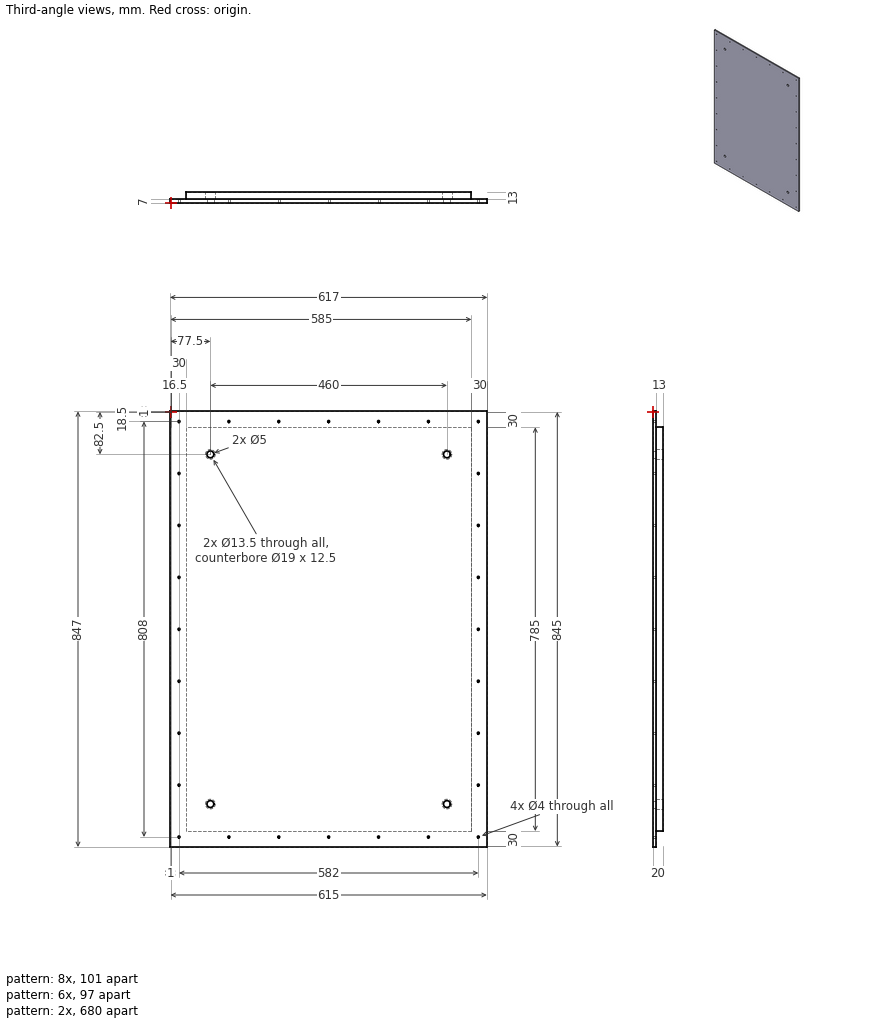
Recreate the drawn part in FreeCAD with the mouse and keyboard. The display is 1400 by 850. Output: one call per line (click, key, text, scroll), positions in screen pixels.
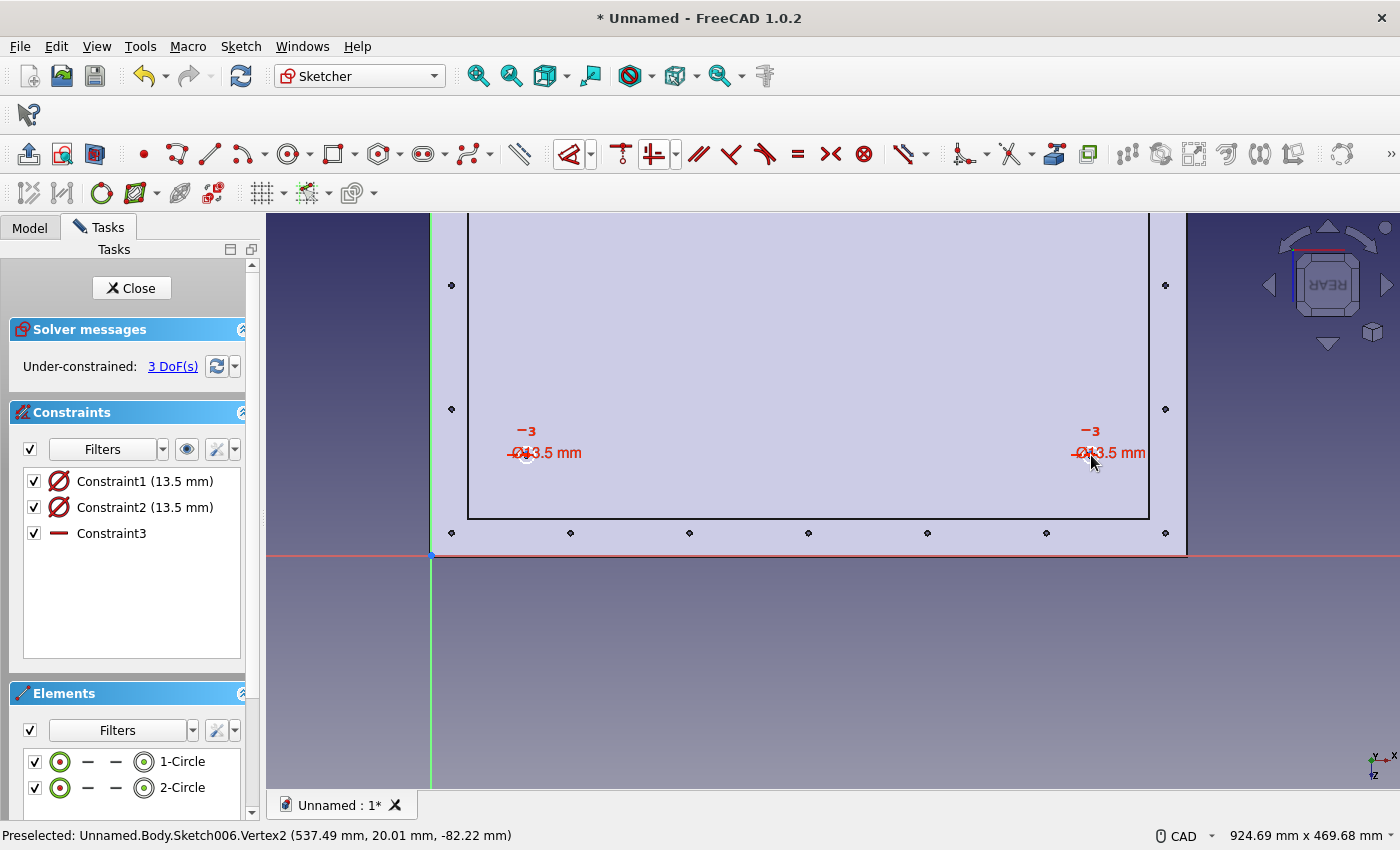
click(527, 455)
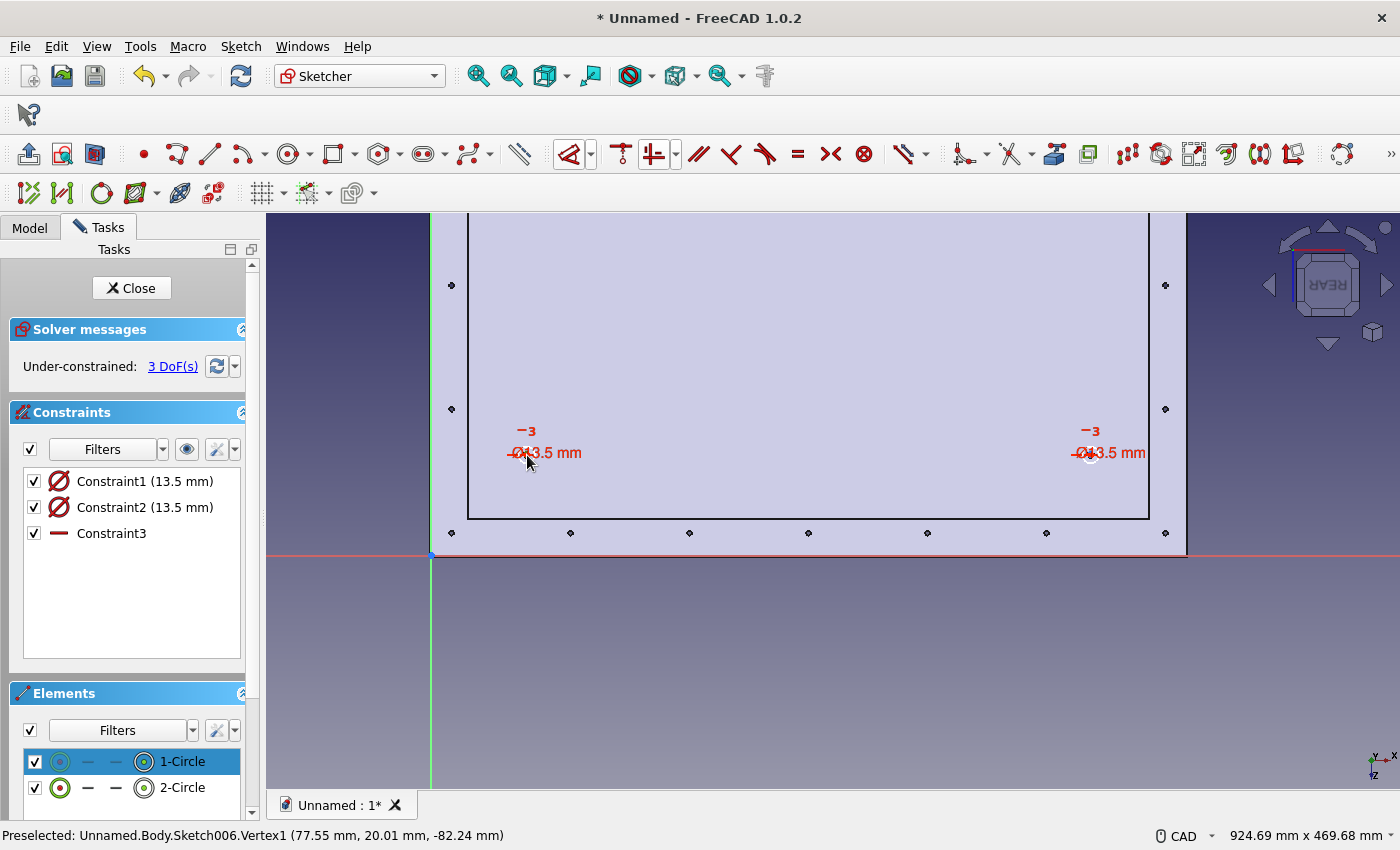
key(l)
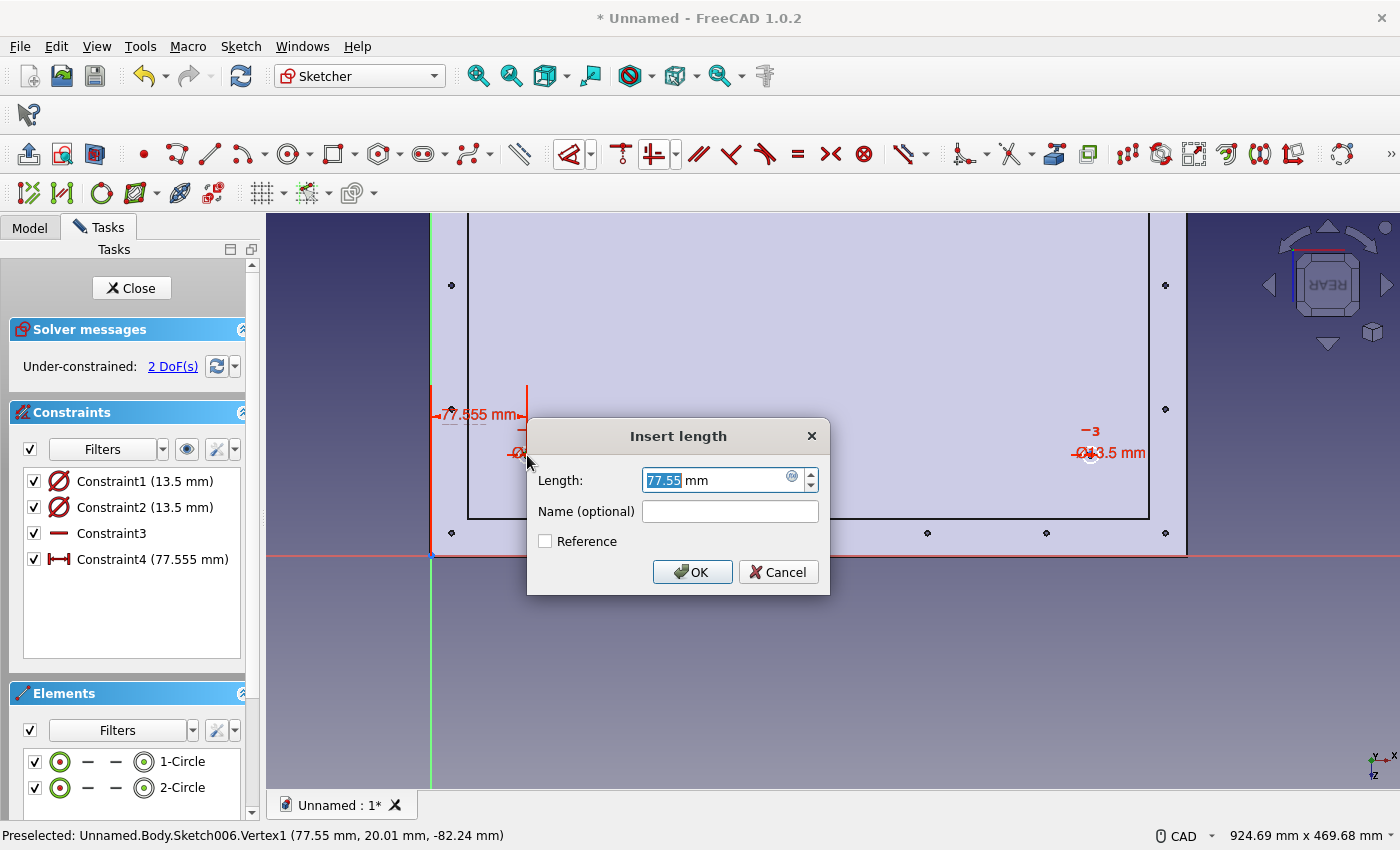
text(77.5)
key(Return)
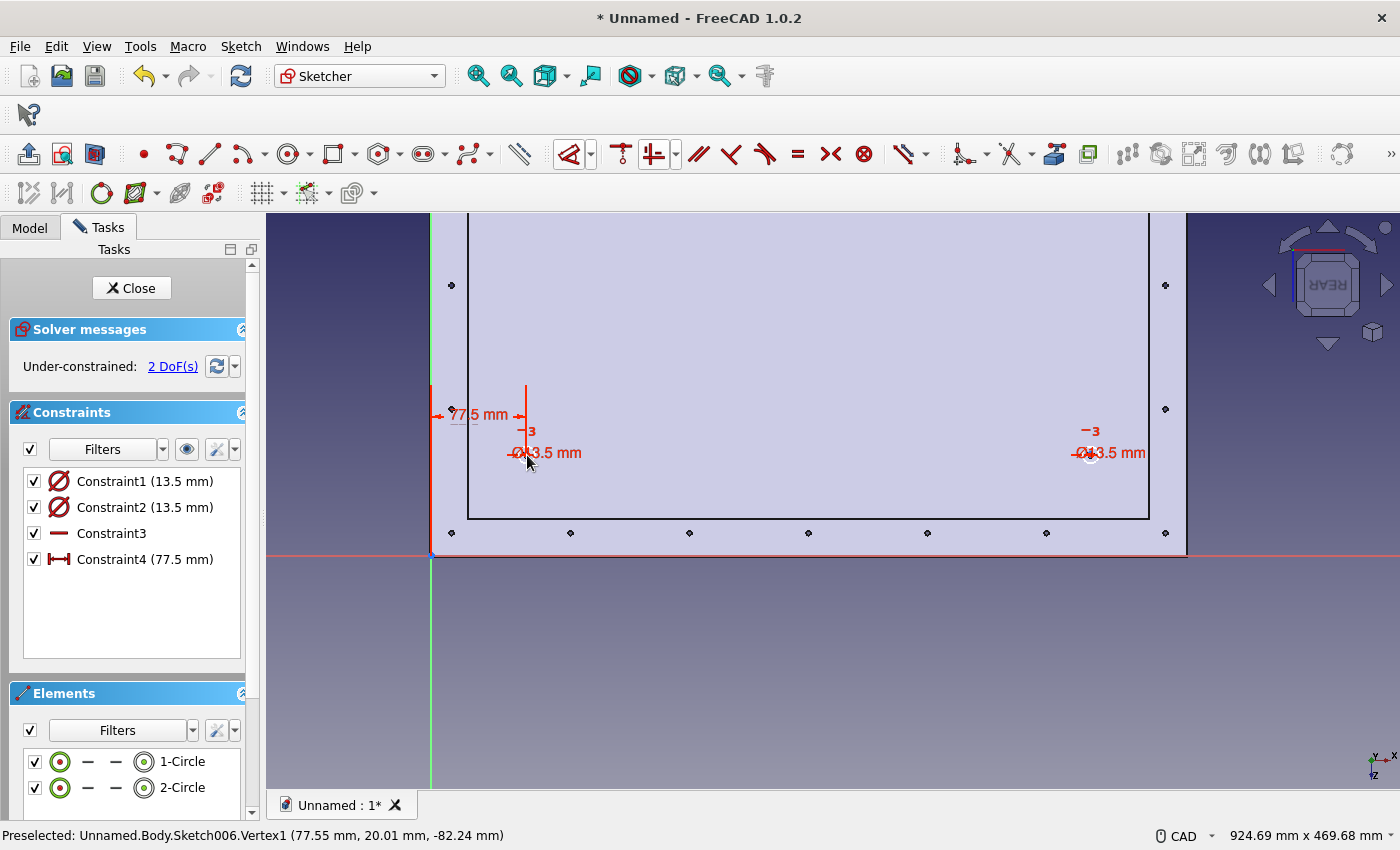
click(526, 455)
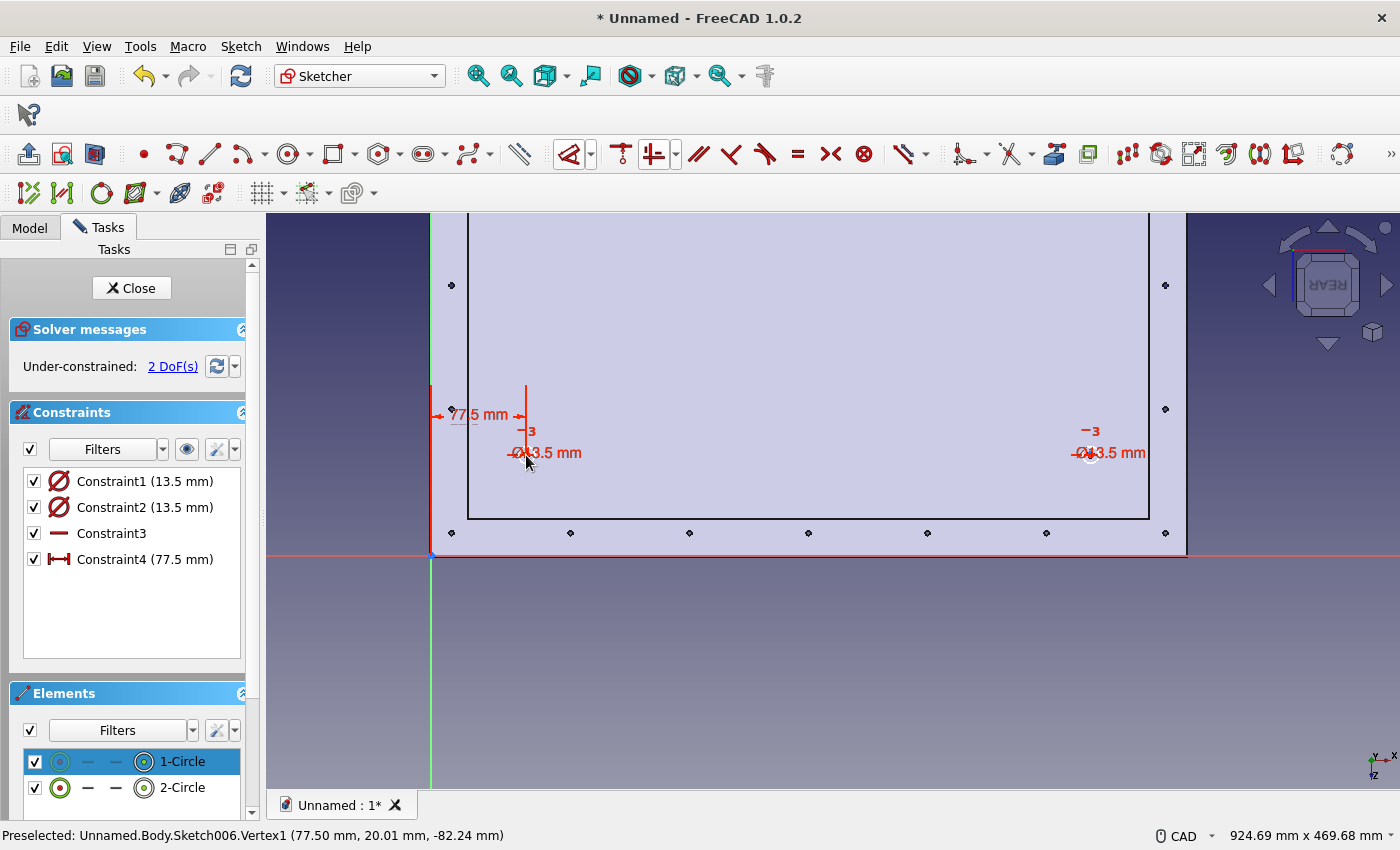
click(590, 154)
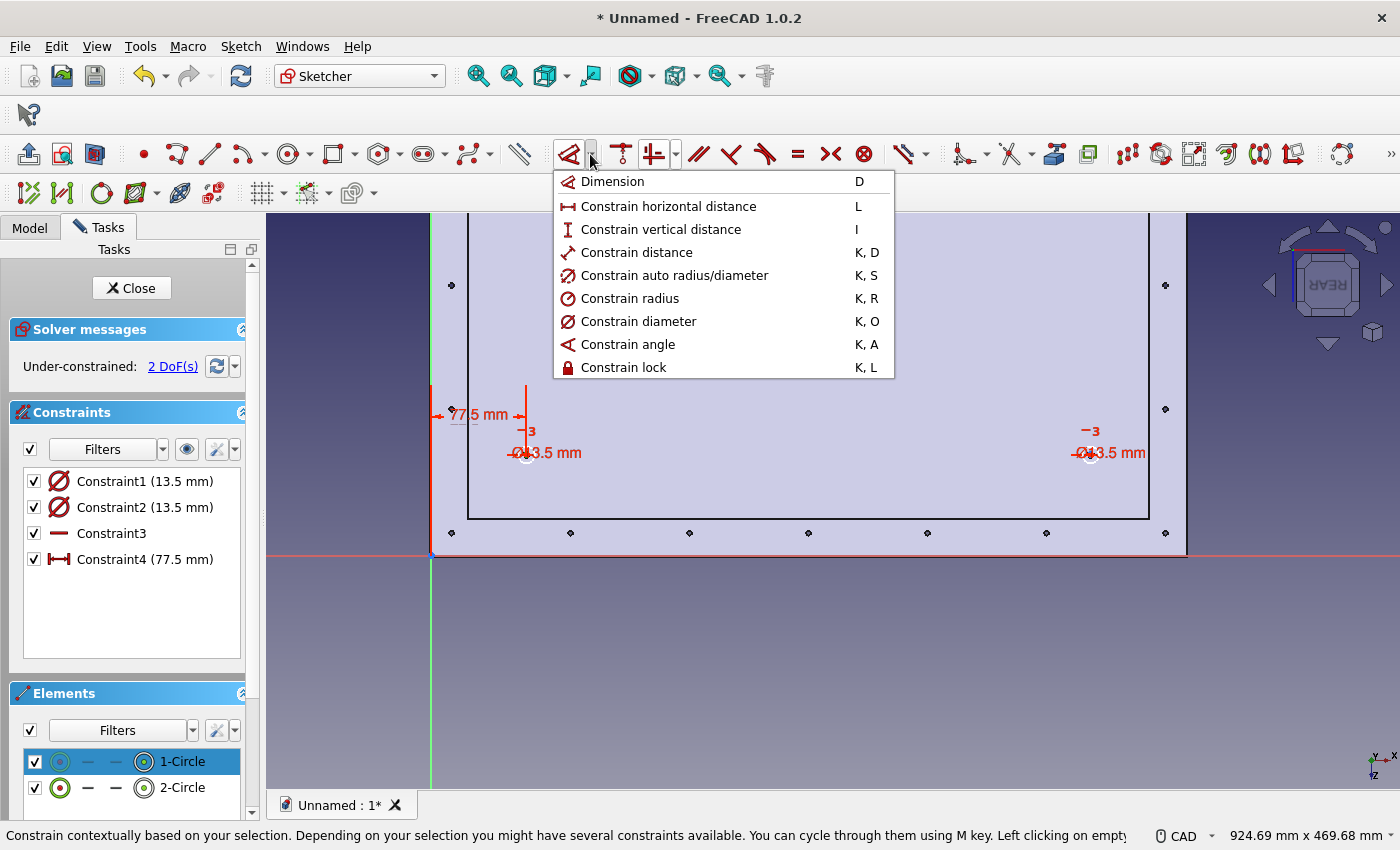
click(724, 230)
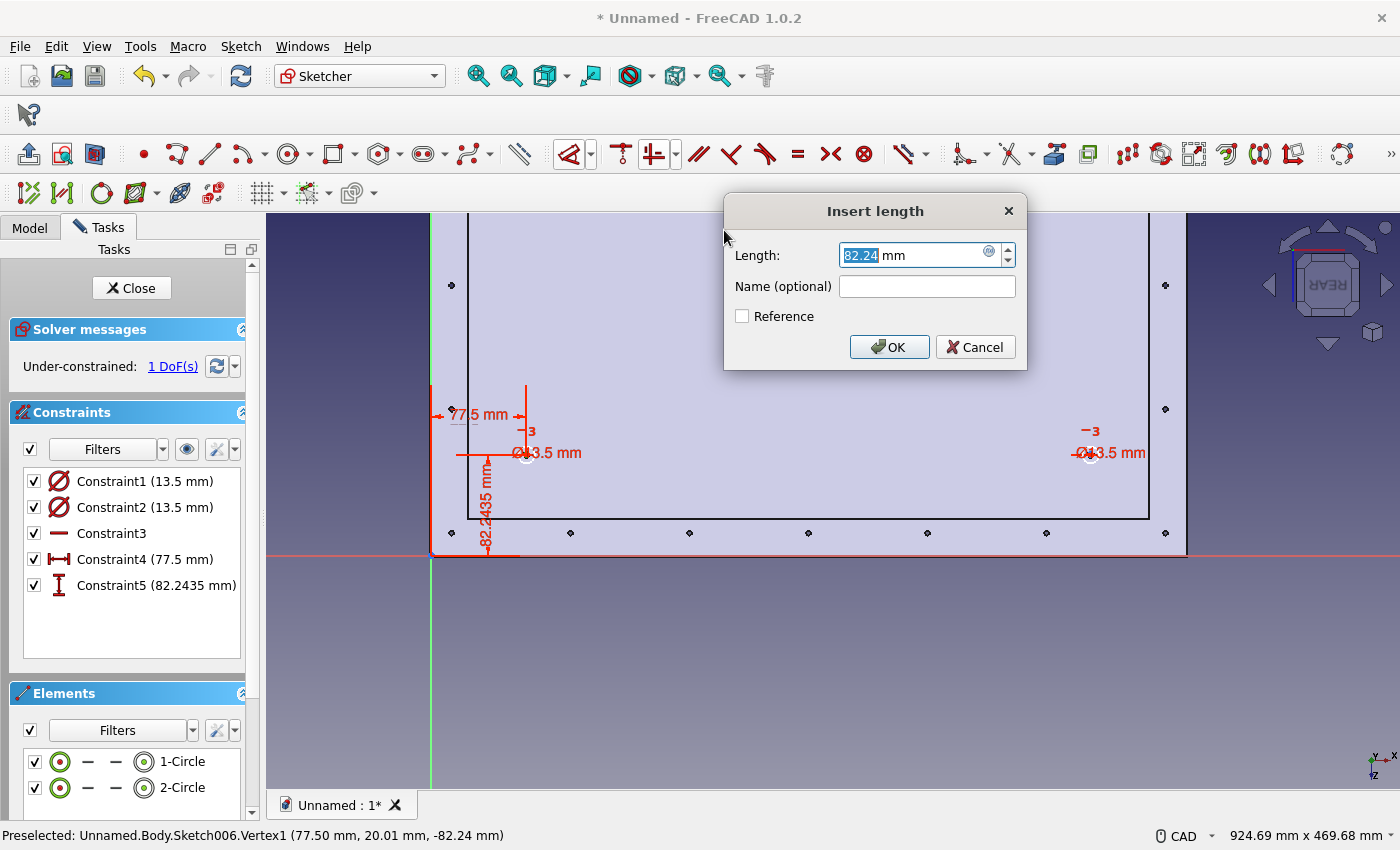
text(82.5)
key(Return)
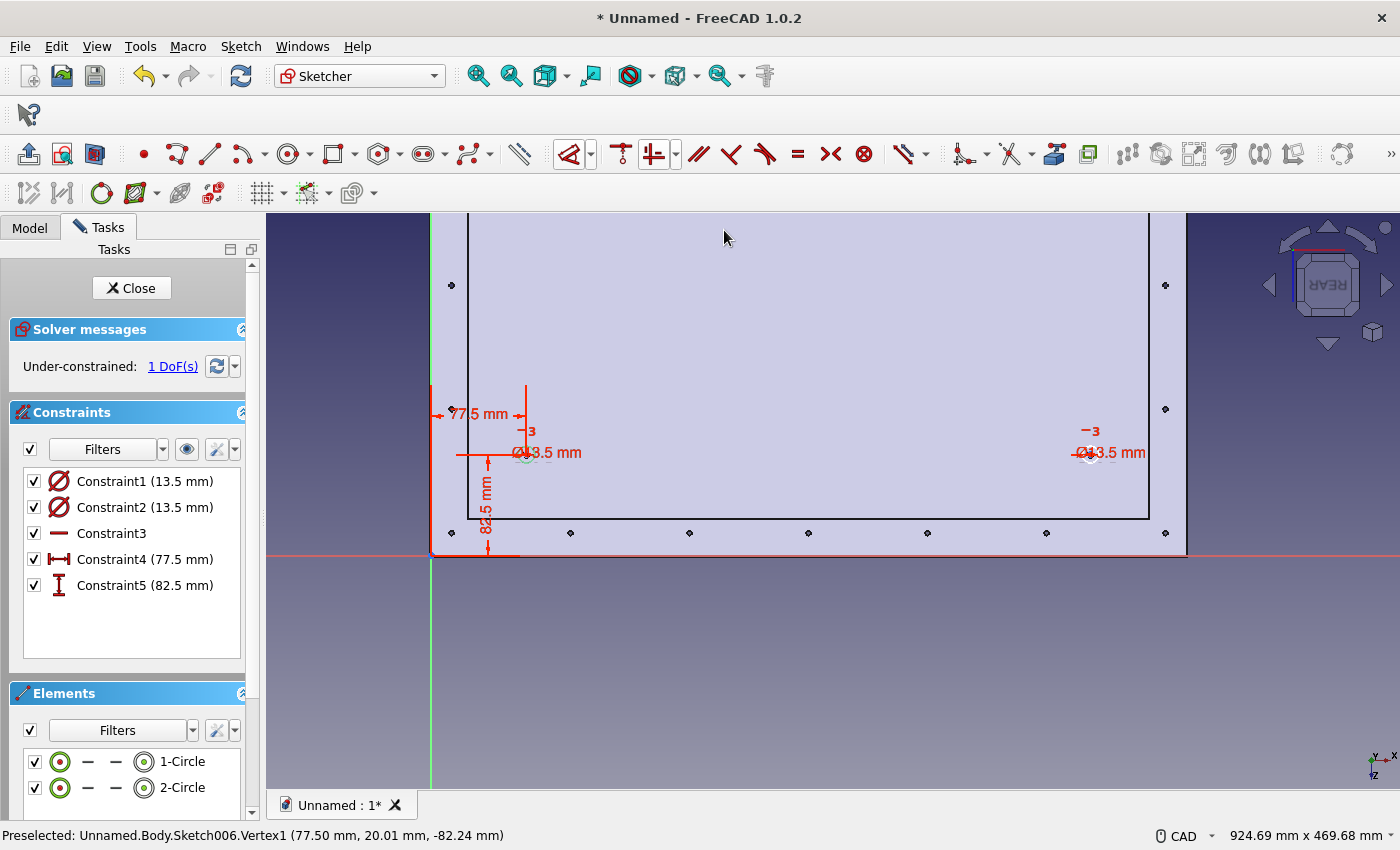
click(526, 455)